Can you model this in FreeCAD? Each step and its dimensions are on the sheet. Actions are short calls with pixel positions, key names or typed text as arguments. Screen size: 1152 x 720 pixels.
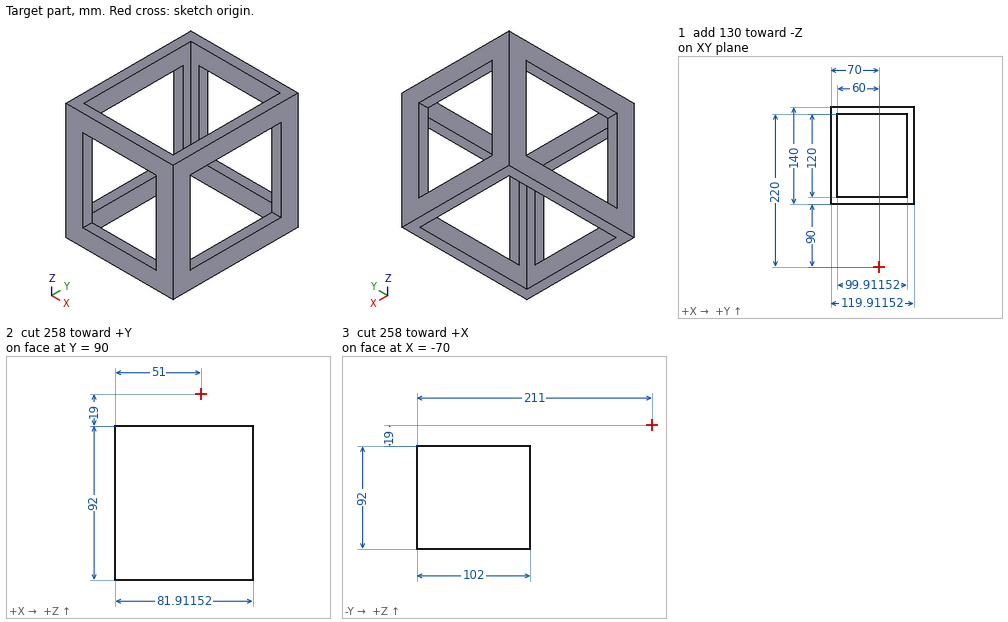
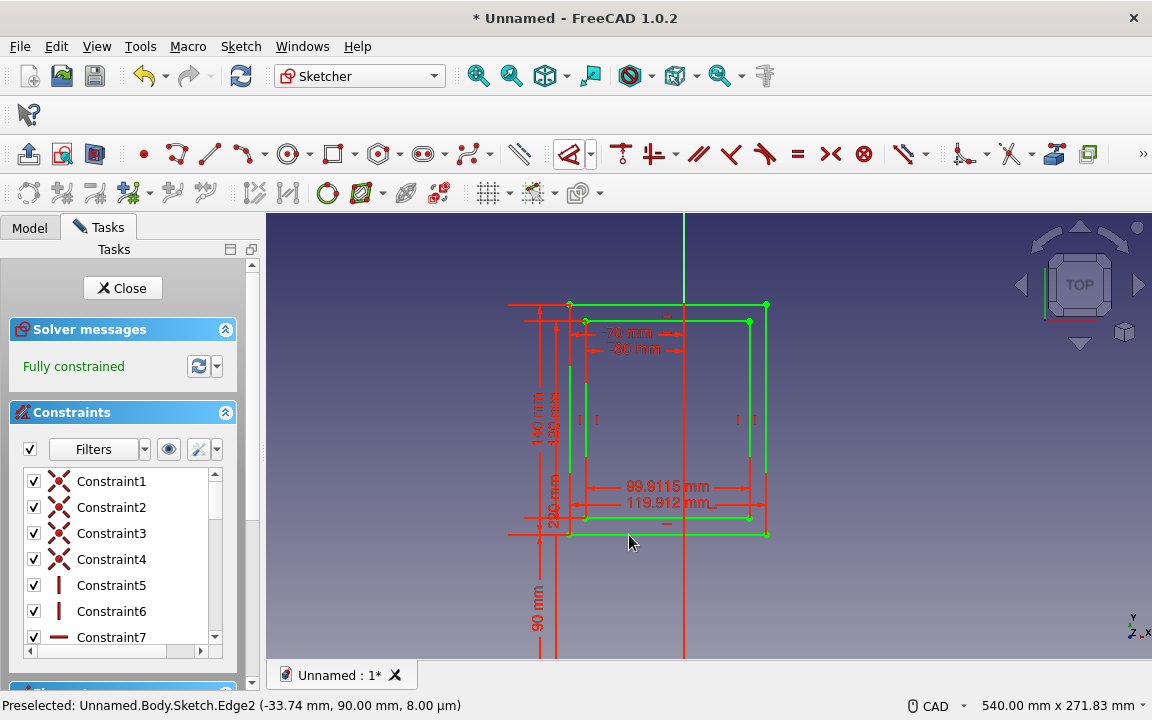
click(123, 288)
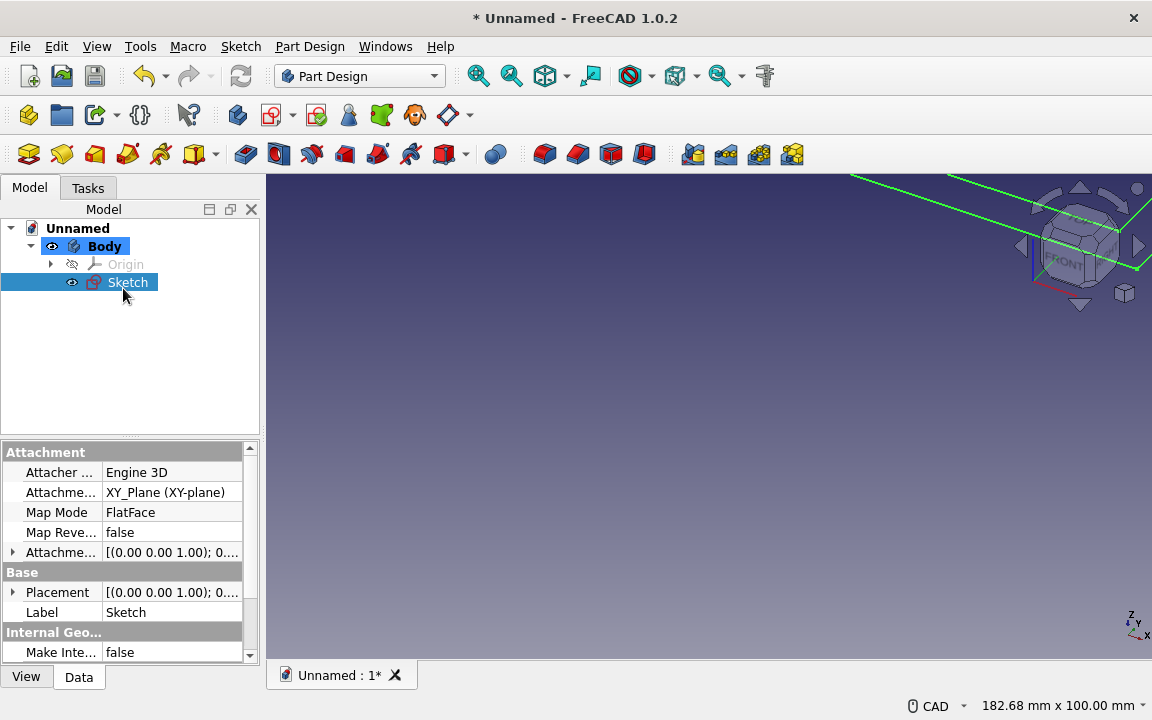
click(29, 154)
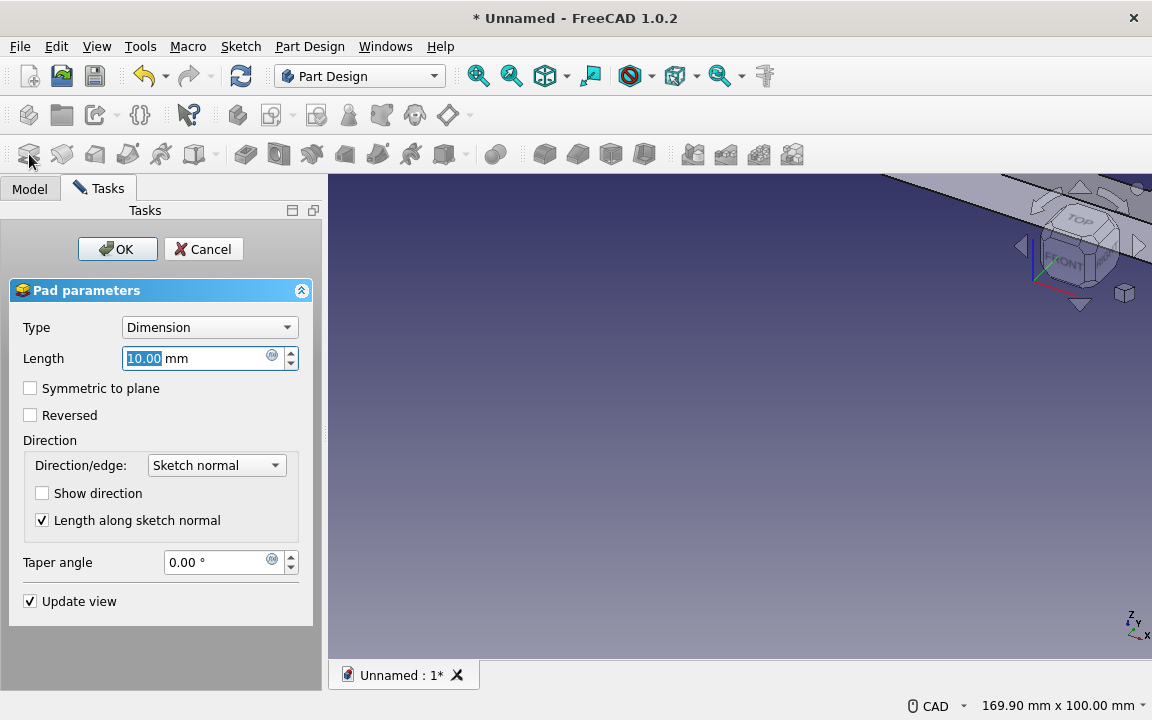
text(130)
key(Tab)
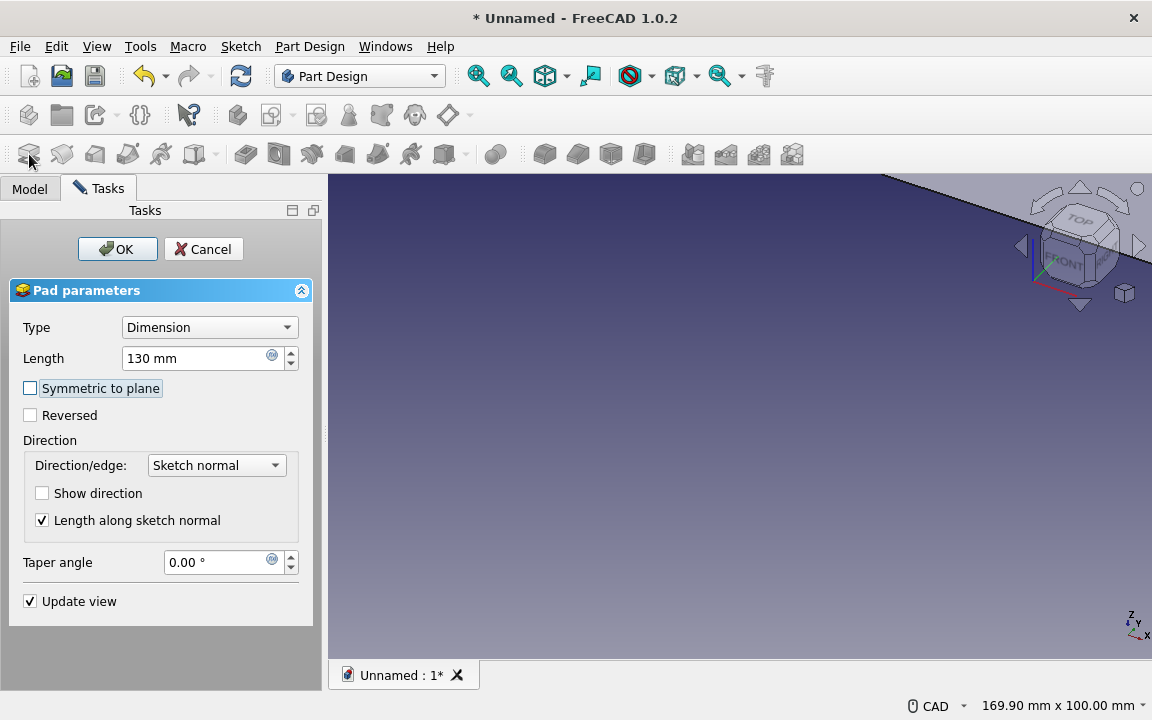
click(31, 415)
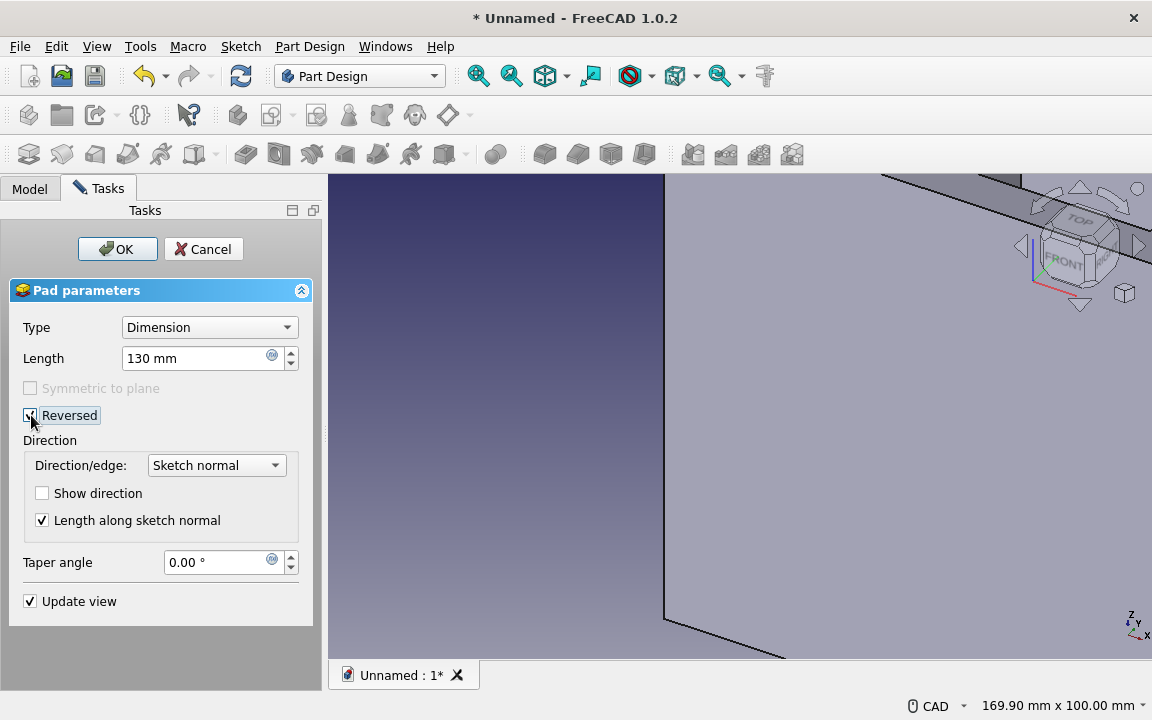
click(118, 249)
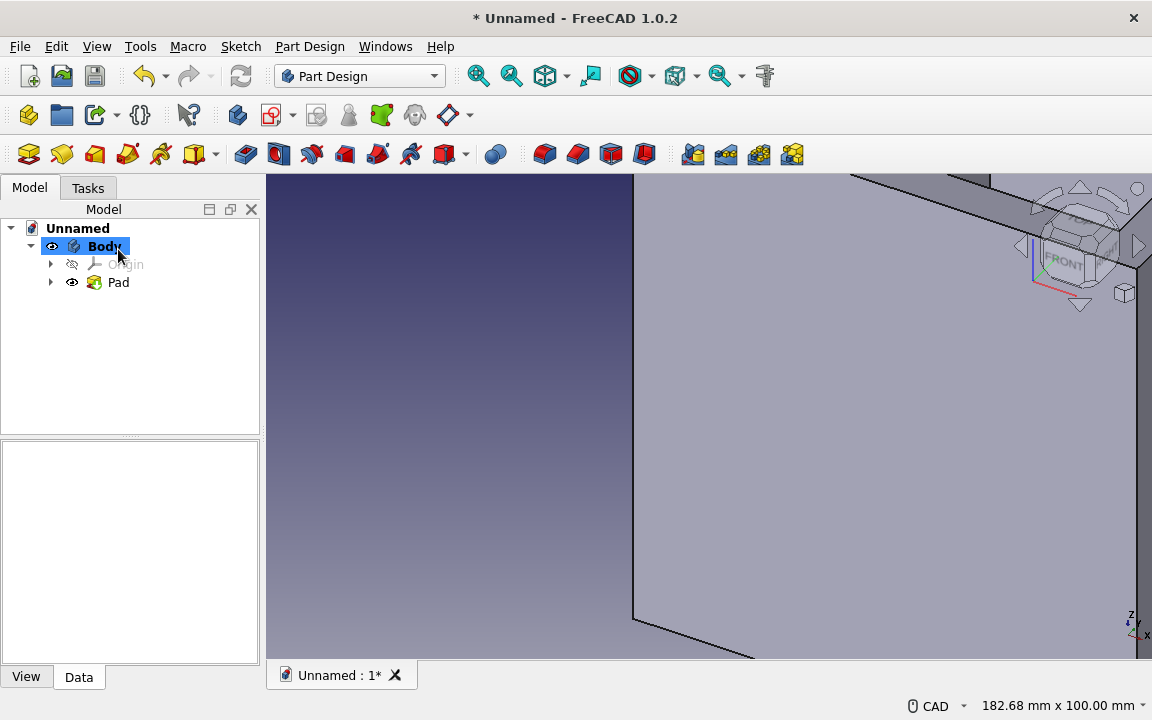
key(v)
key(f)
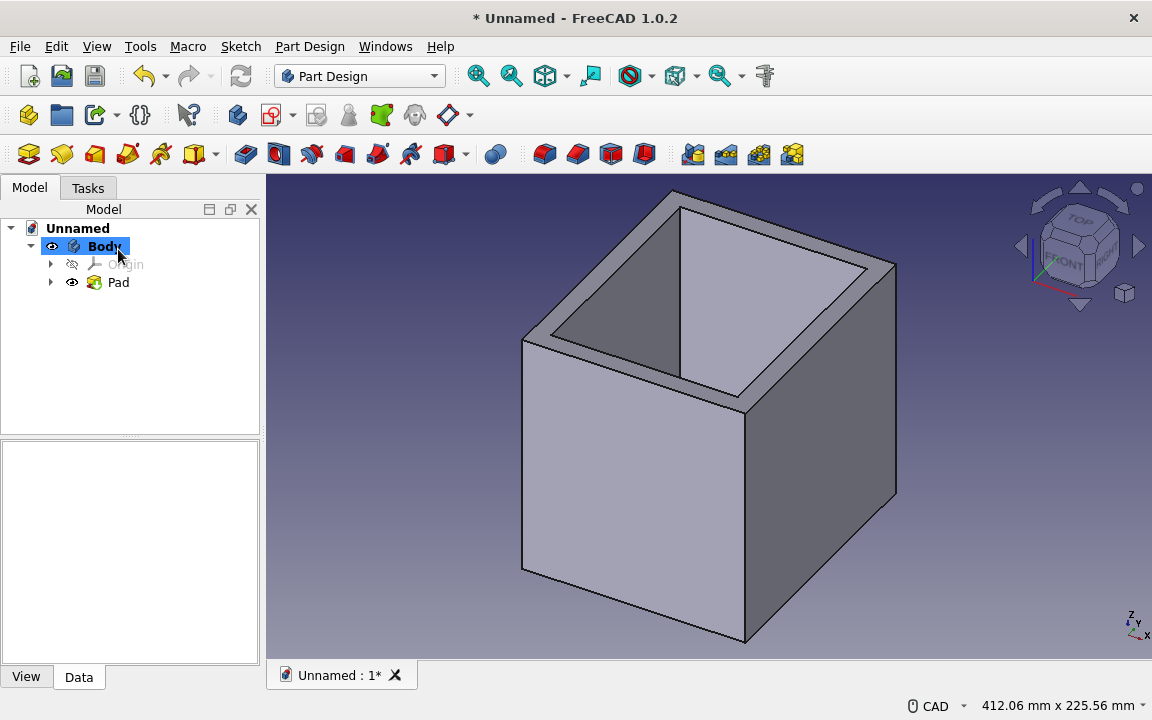
click(634, 490)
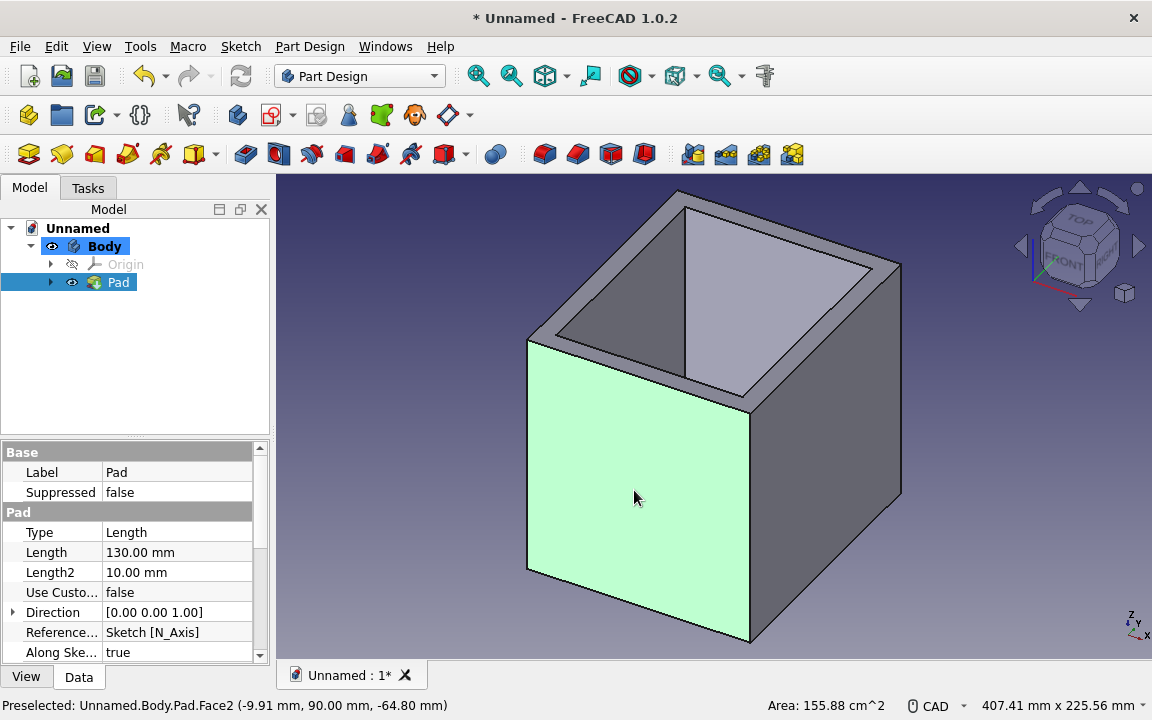
click(270, 116)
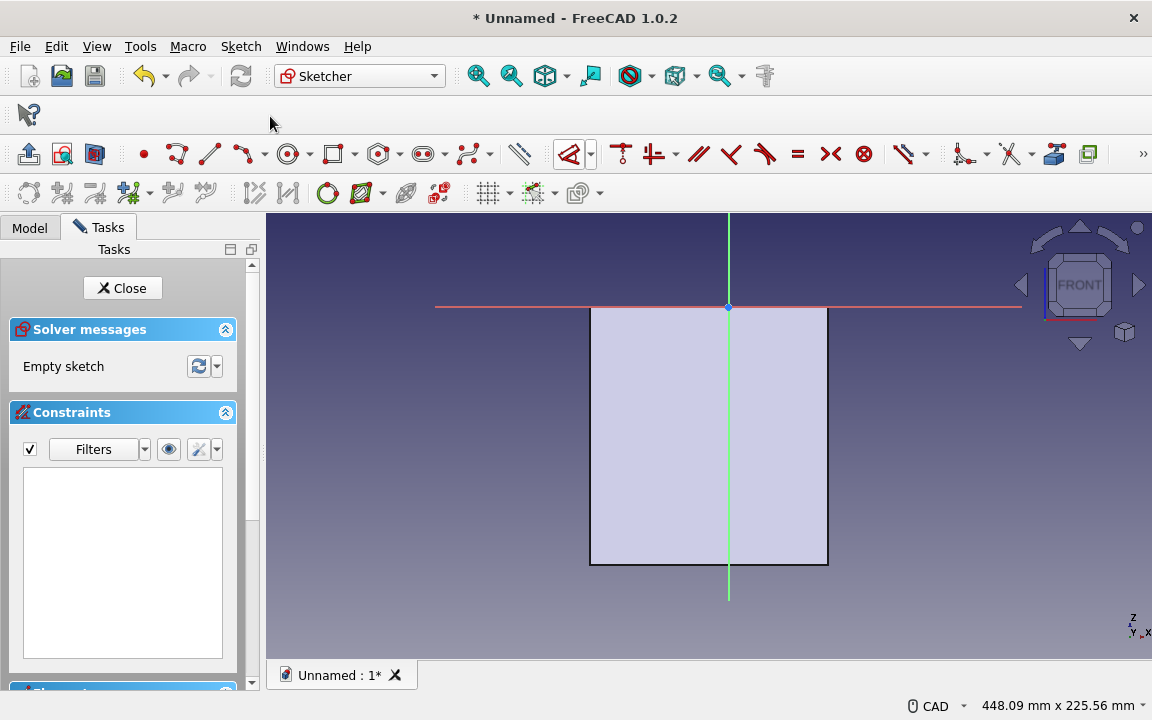
key(g)
key(r)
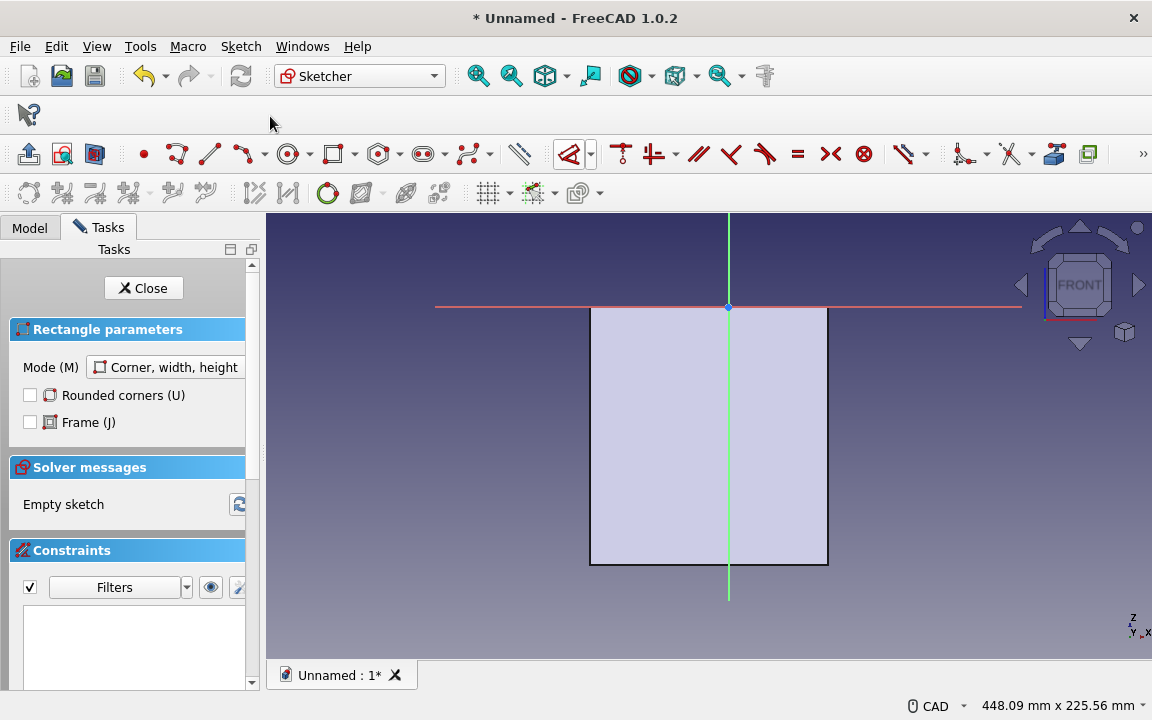
click(628, 345)
click(790, 527)
key(Escape)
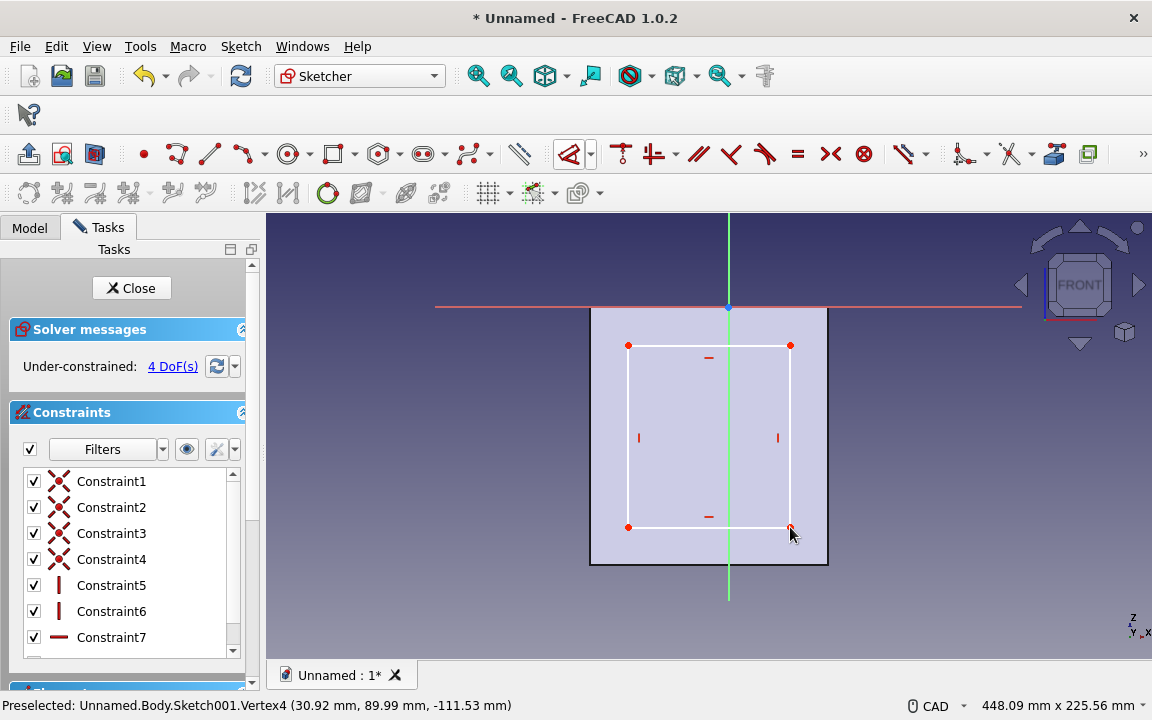
click(628, 401)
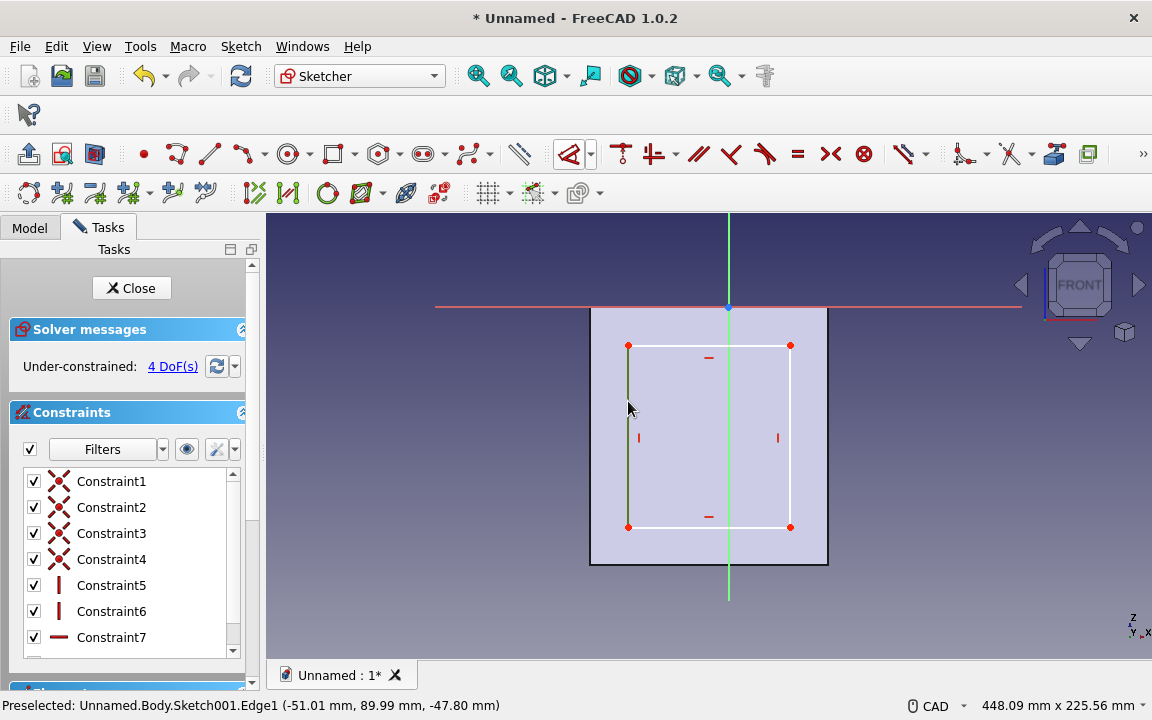
key(i)